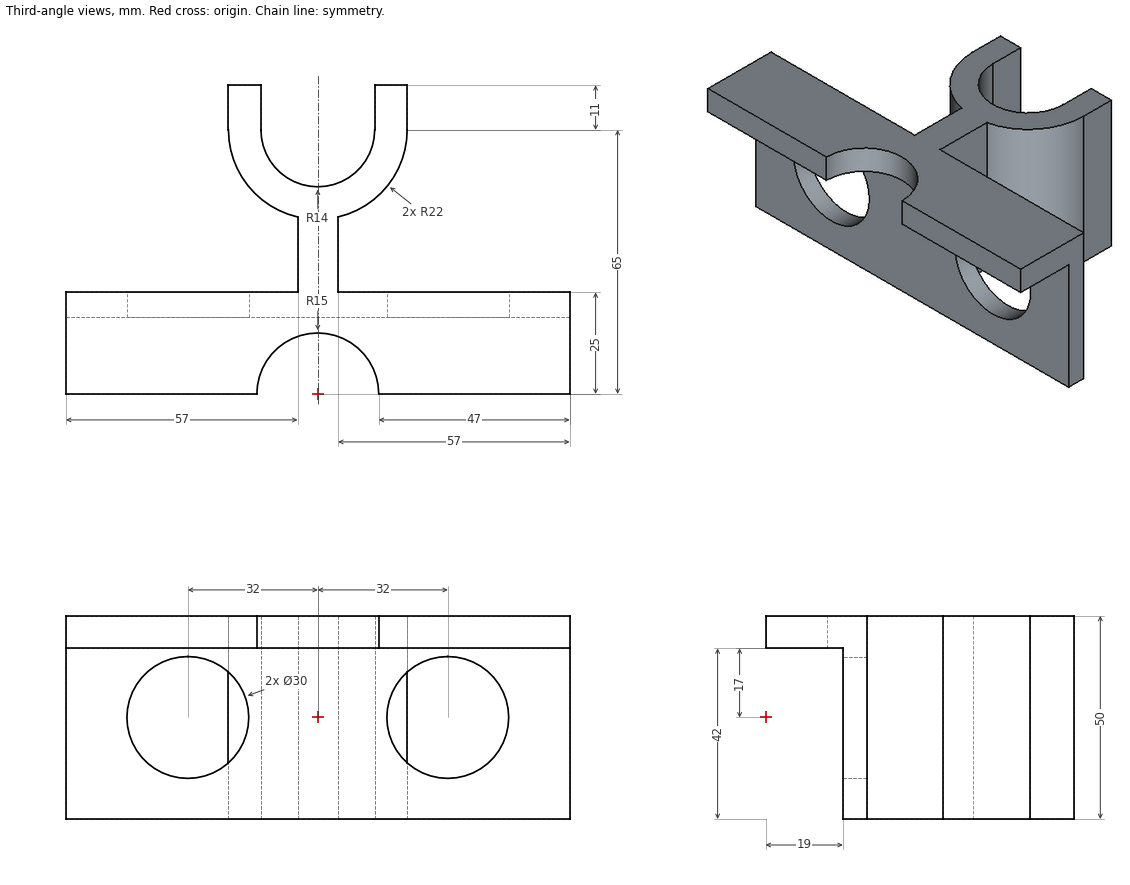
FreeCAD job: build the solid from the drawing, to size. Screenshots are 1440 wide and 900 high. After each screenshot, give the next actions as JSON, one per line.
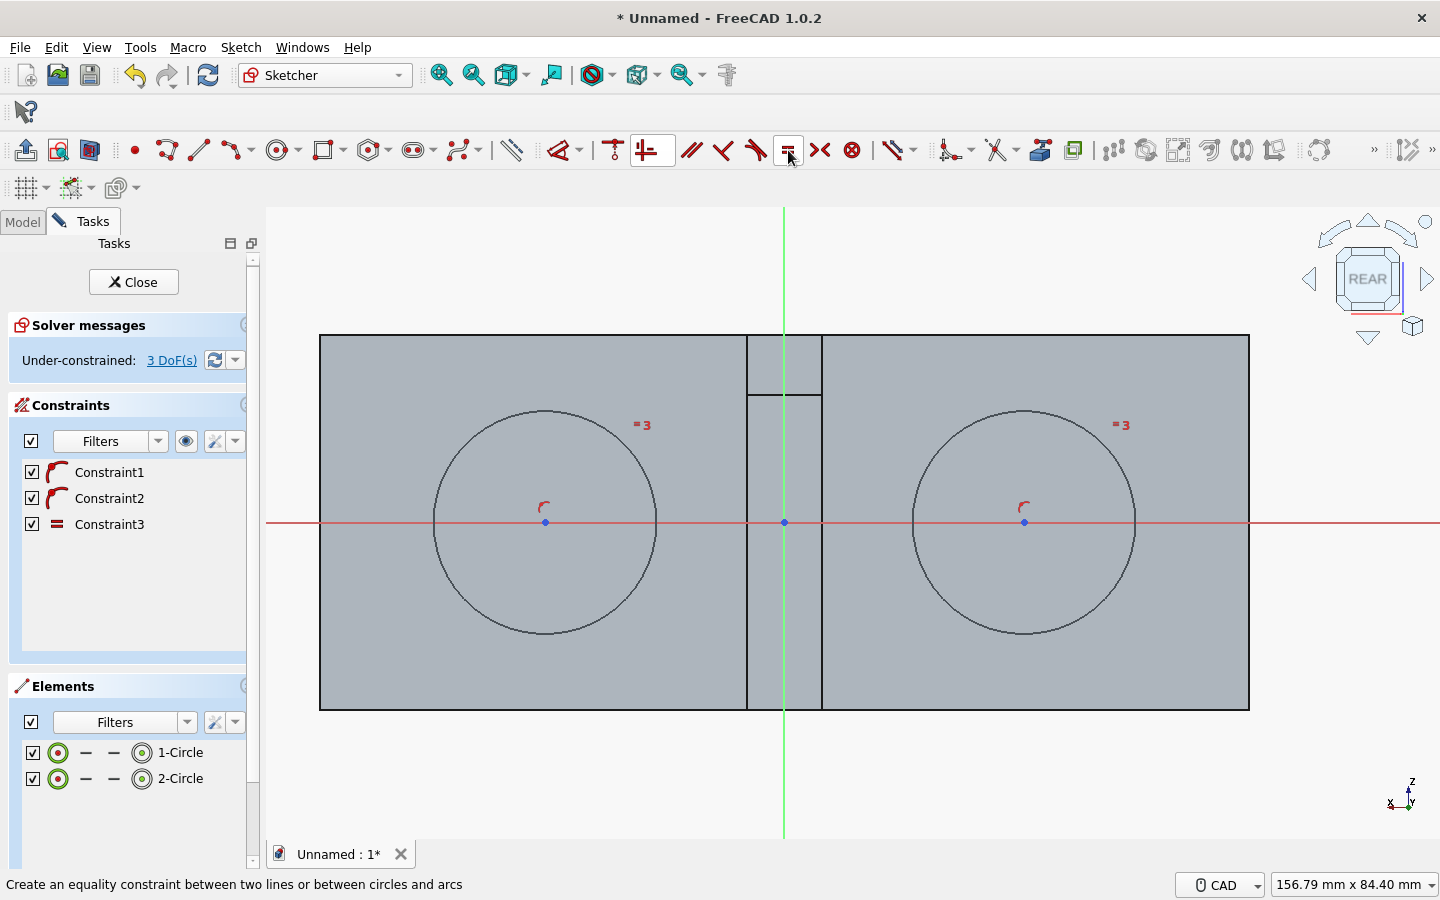
{"action": "left_click", "coordinate": [558, 150]}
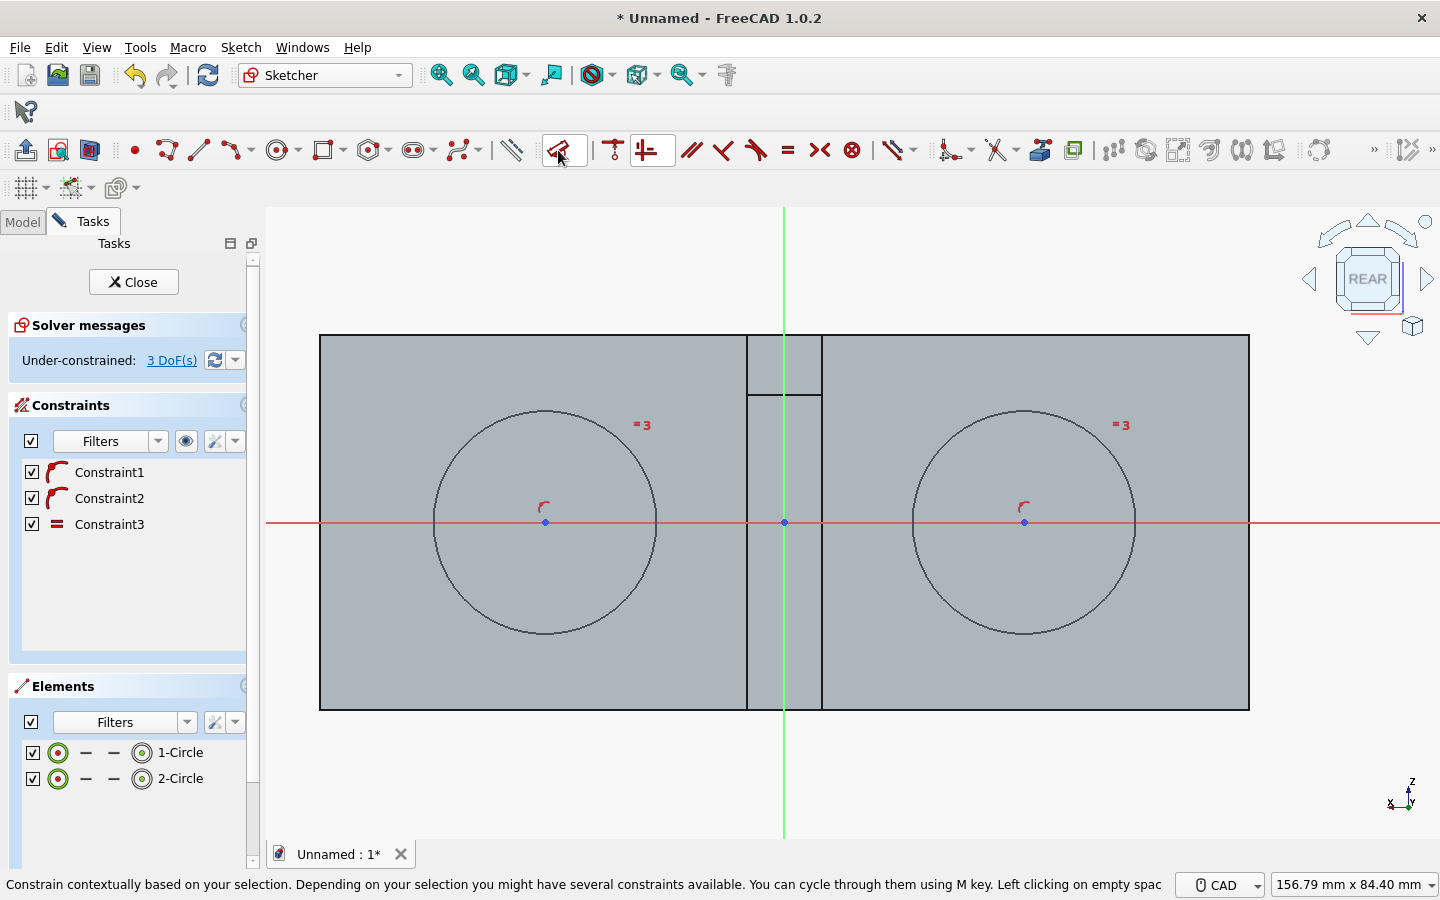
{"action": "left_click", "coordinate": [1103, 444]}
{"action": "left_click", "coordinate": [1126, 421]}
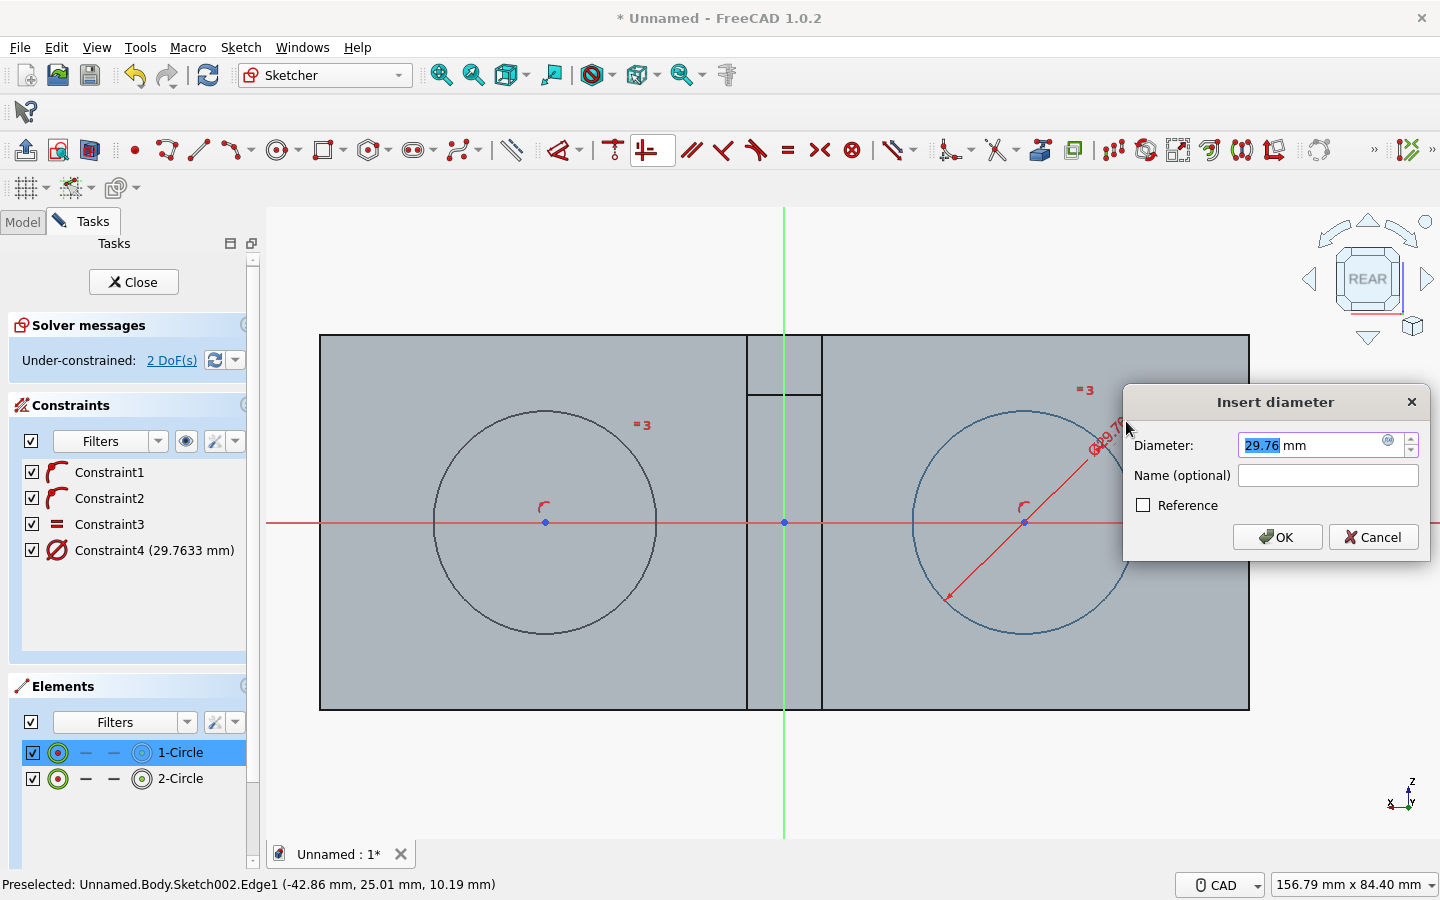
{"action": "type", "text": "30"}
{"action": "key", "text": "Return"}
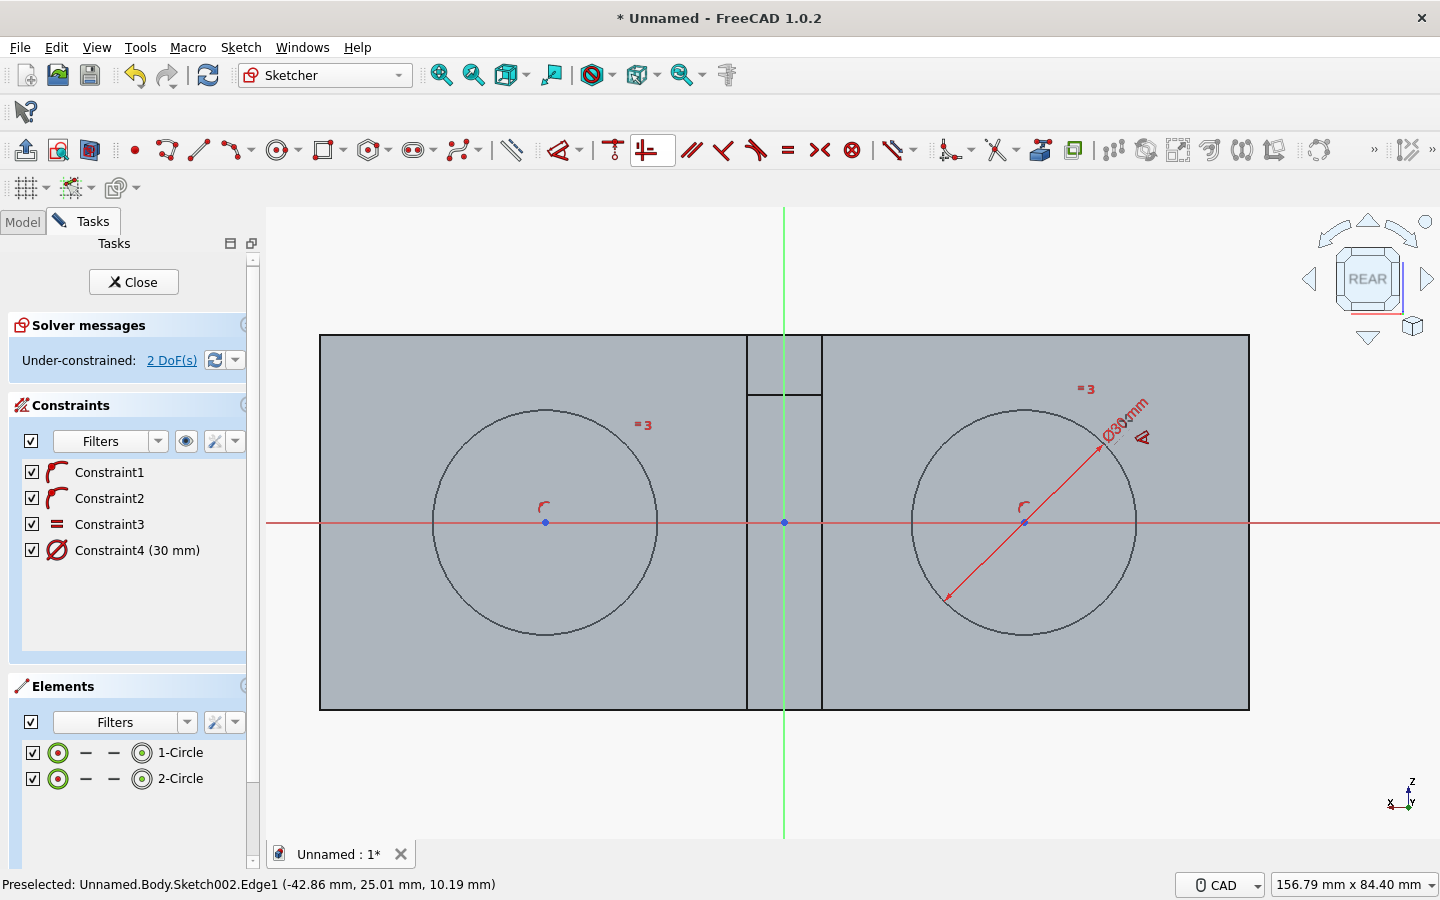
{"action": "left_click", "coordinate": [1024, 523]}
{"action": "left_click", "coordinate": [849, 557]}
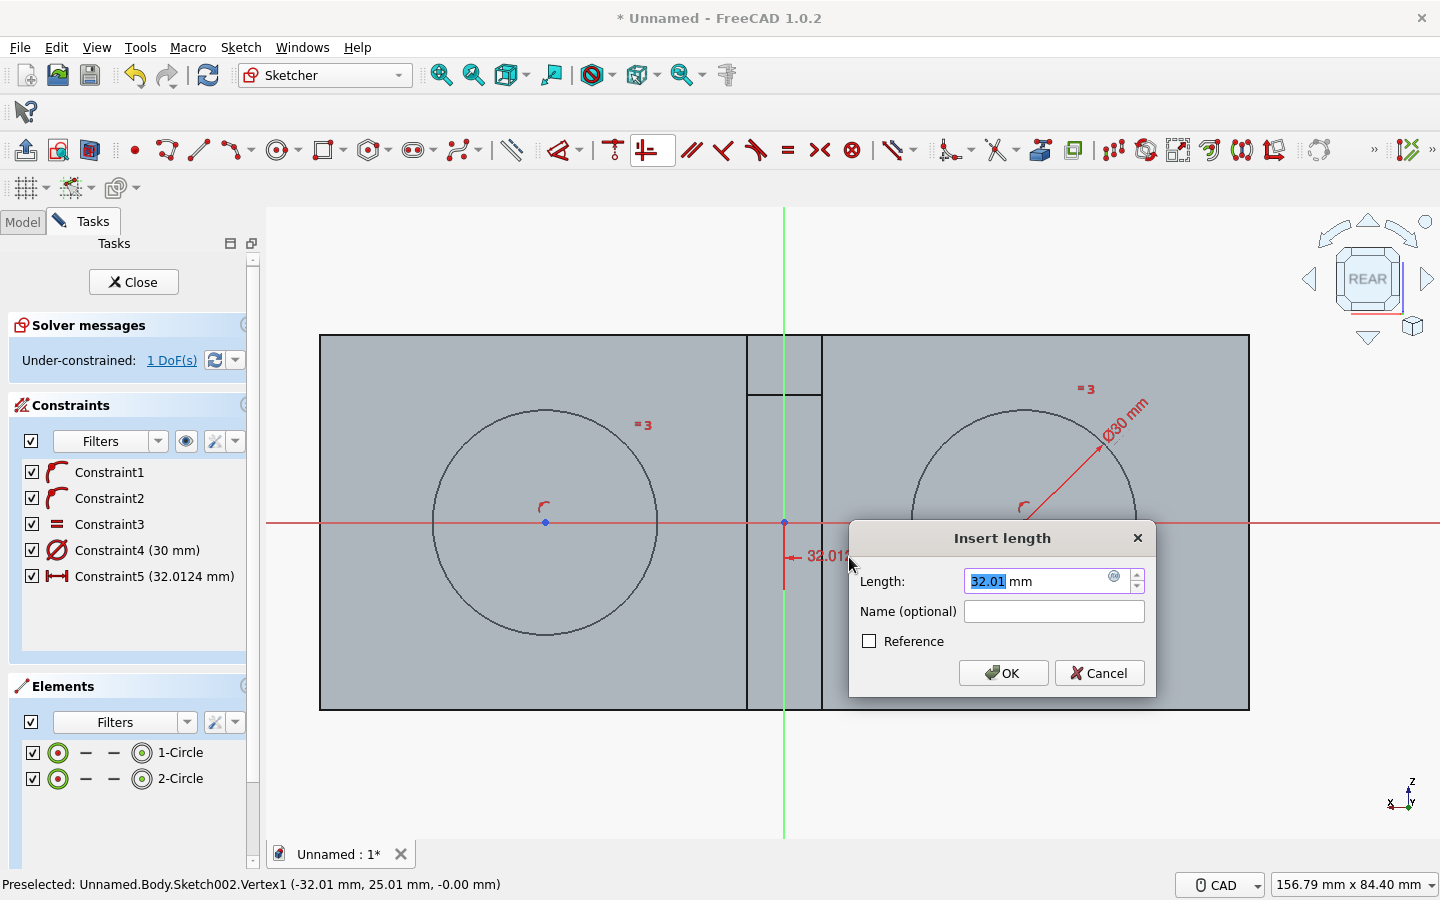
{"action": "type", "text": "32"}
{"action": "key", "text": "Return"}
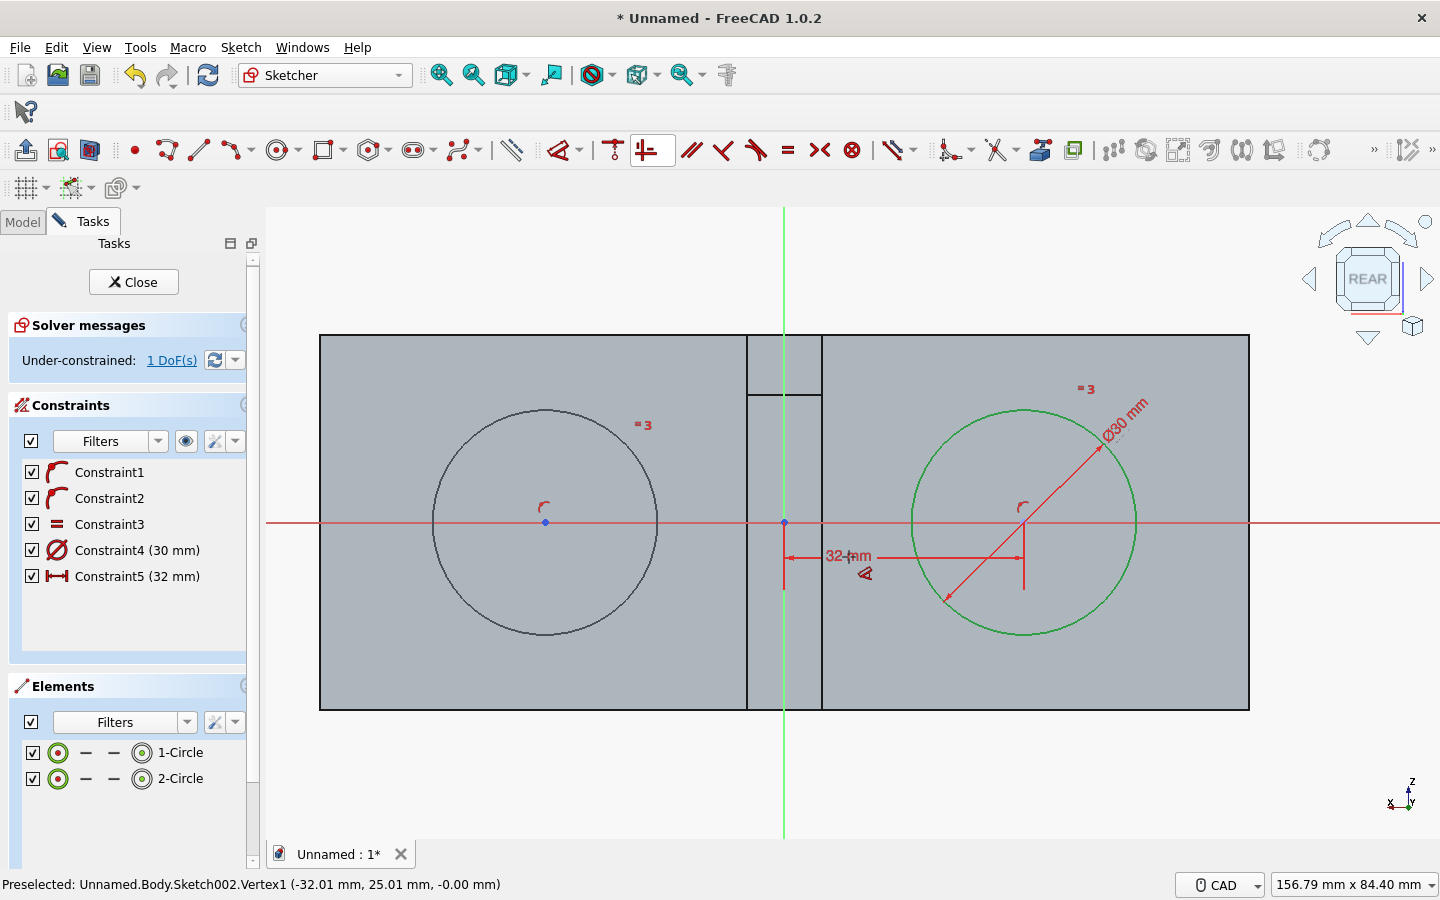
{"action": "left_click", "coordinate": [545, 523]}
{"action": "left_click", "coordinate": [610, 557]}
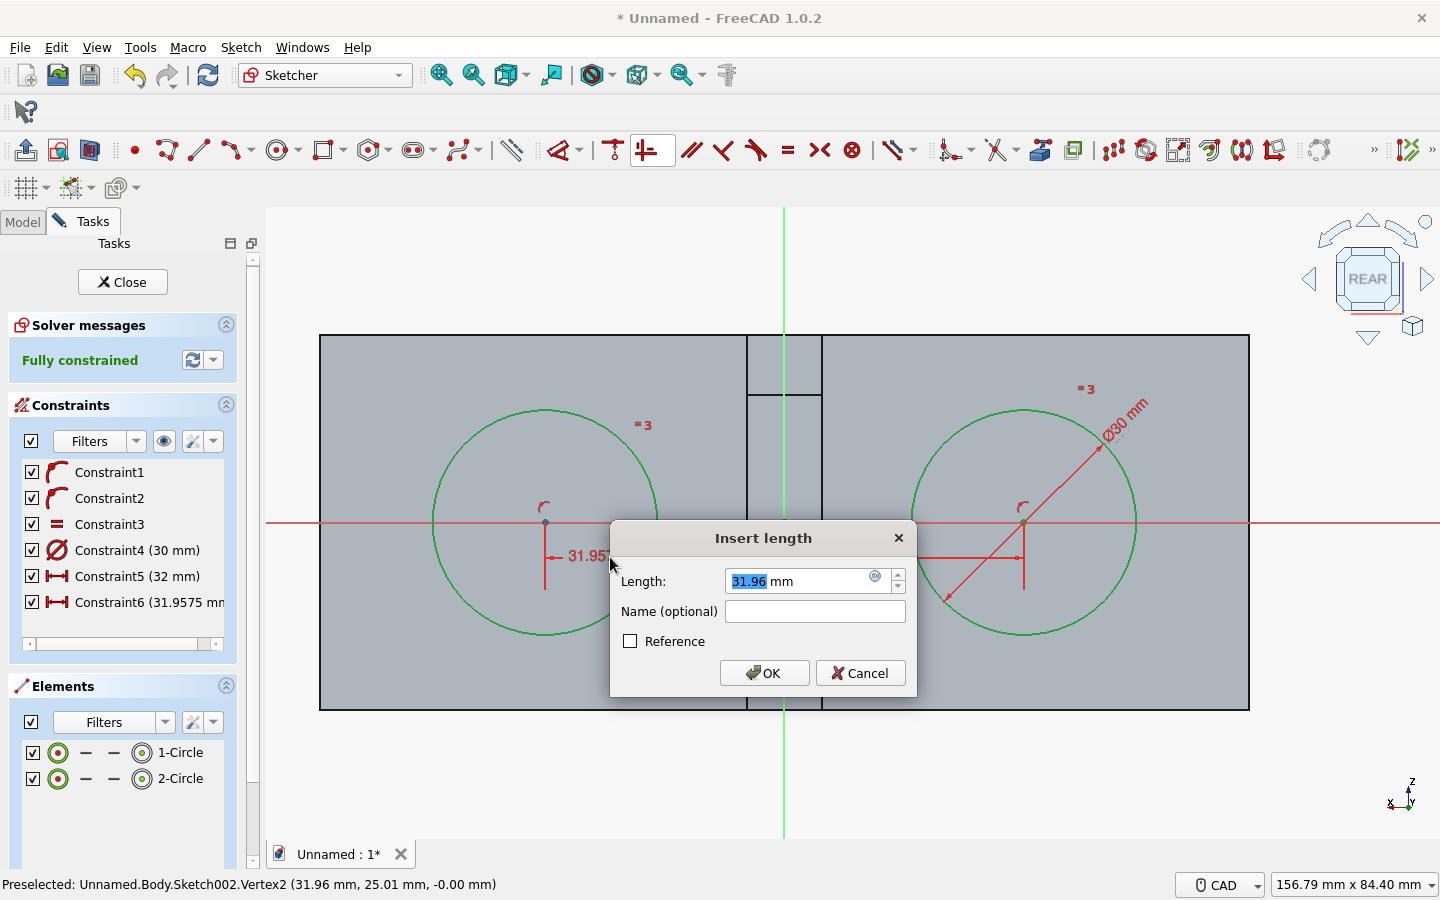
{"action": "type", "text": "32"}
{"action": "key", "text": "Return"}
{"action": "key", "text": "Escape"}